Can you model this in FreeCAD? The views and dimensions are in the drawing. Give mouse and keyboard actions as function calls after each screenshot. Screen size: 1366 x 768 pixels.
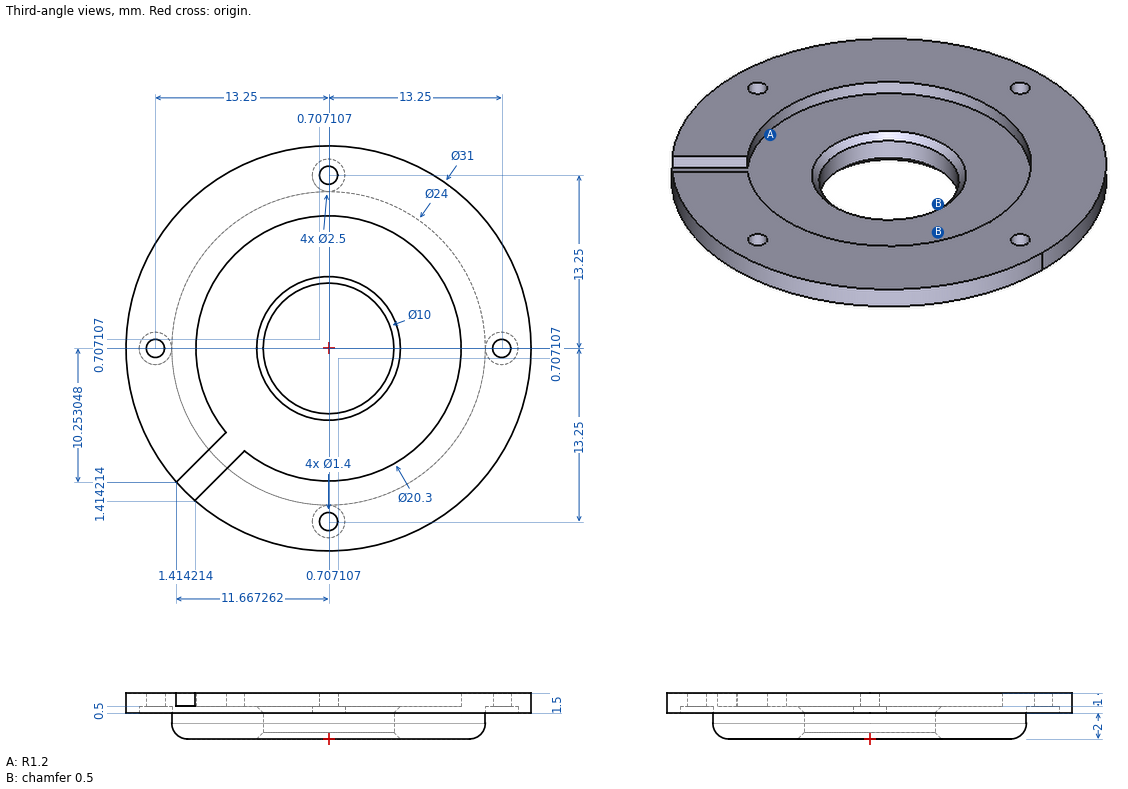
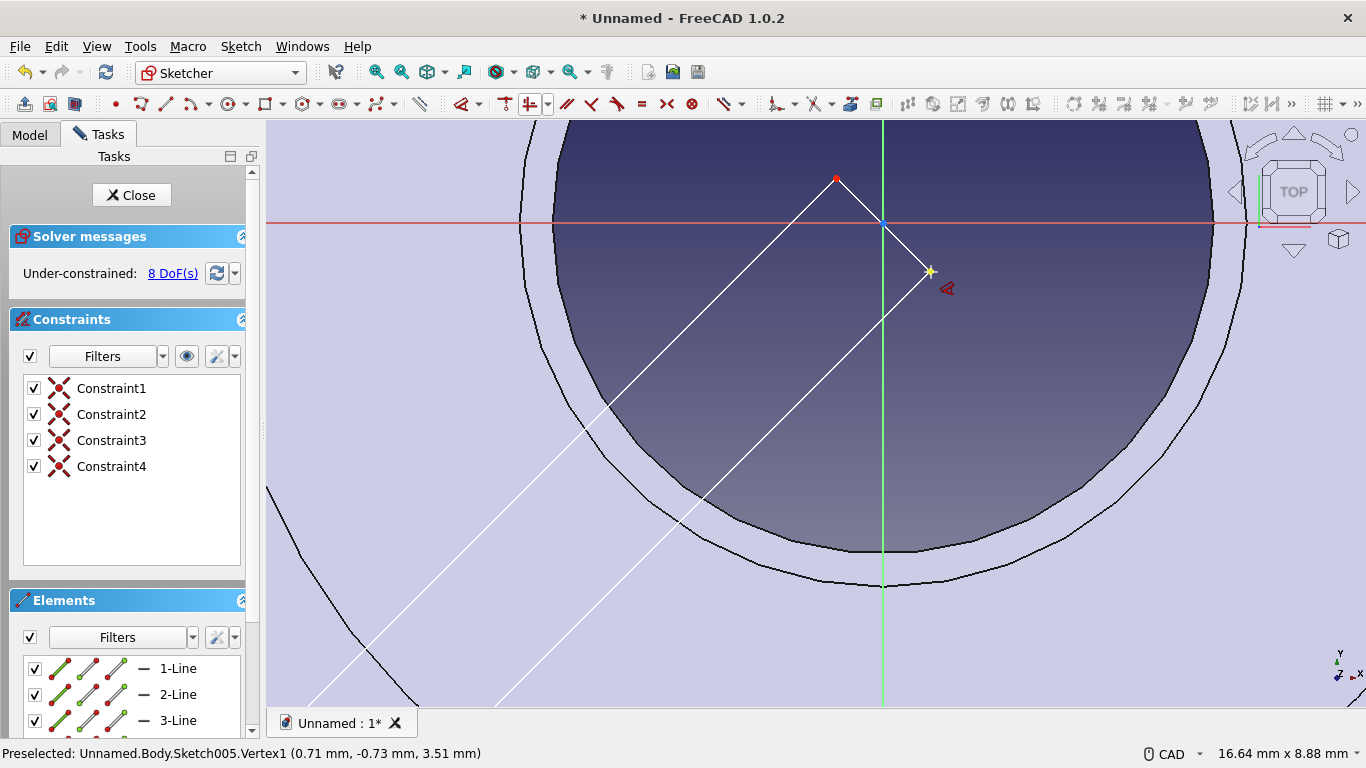
click(930, 272)
click(907, 189)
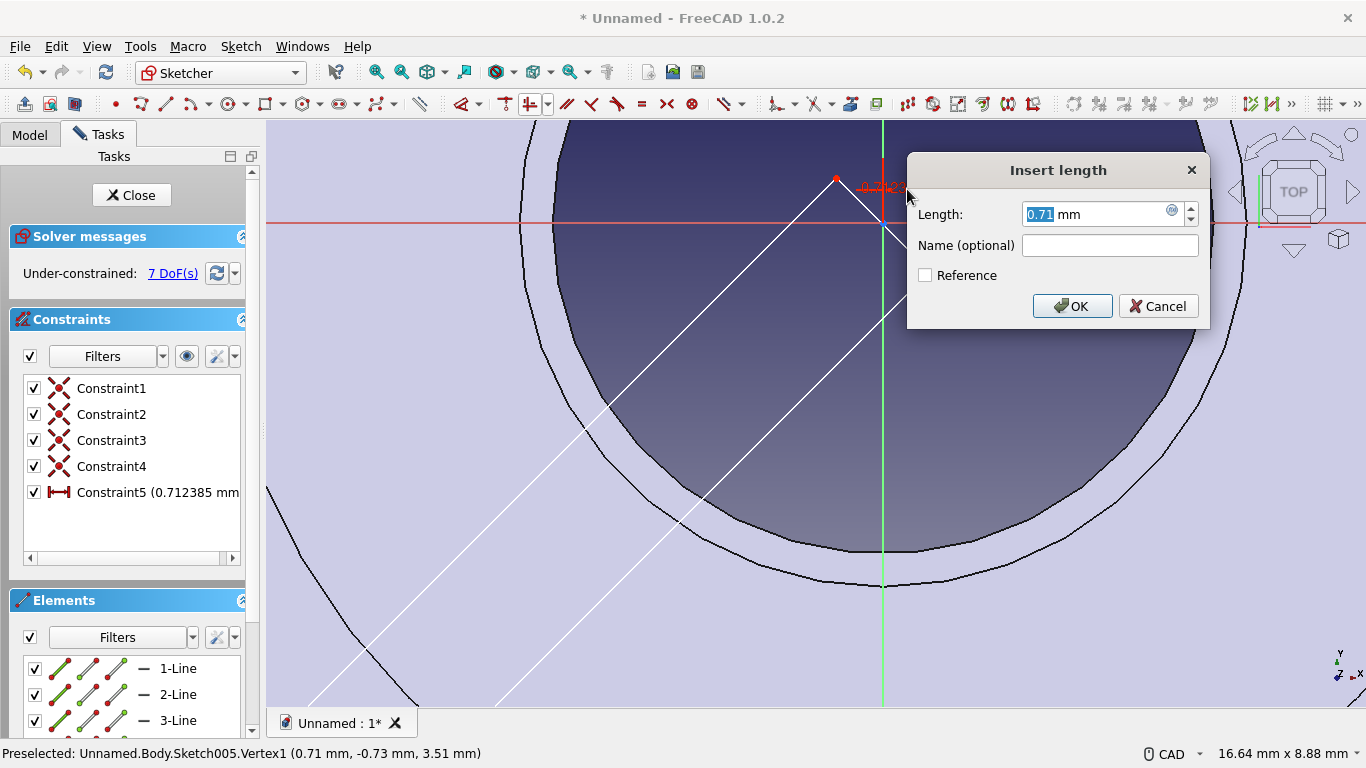
text(0.707107)
key(Return)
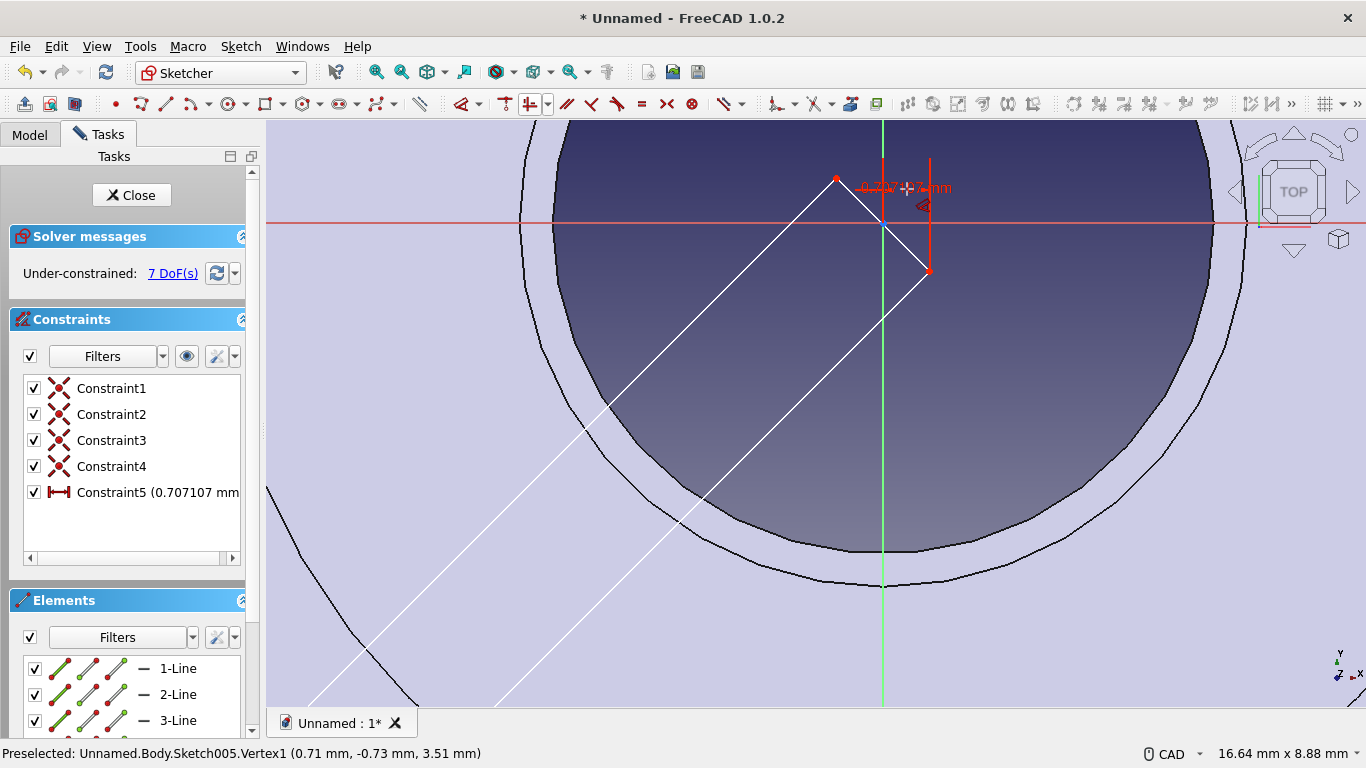
click(930, 272)
click(964, 247)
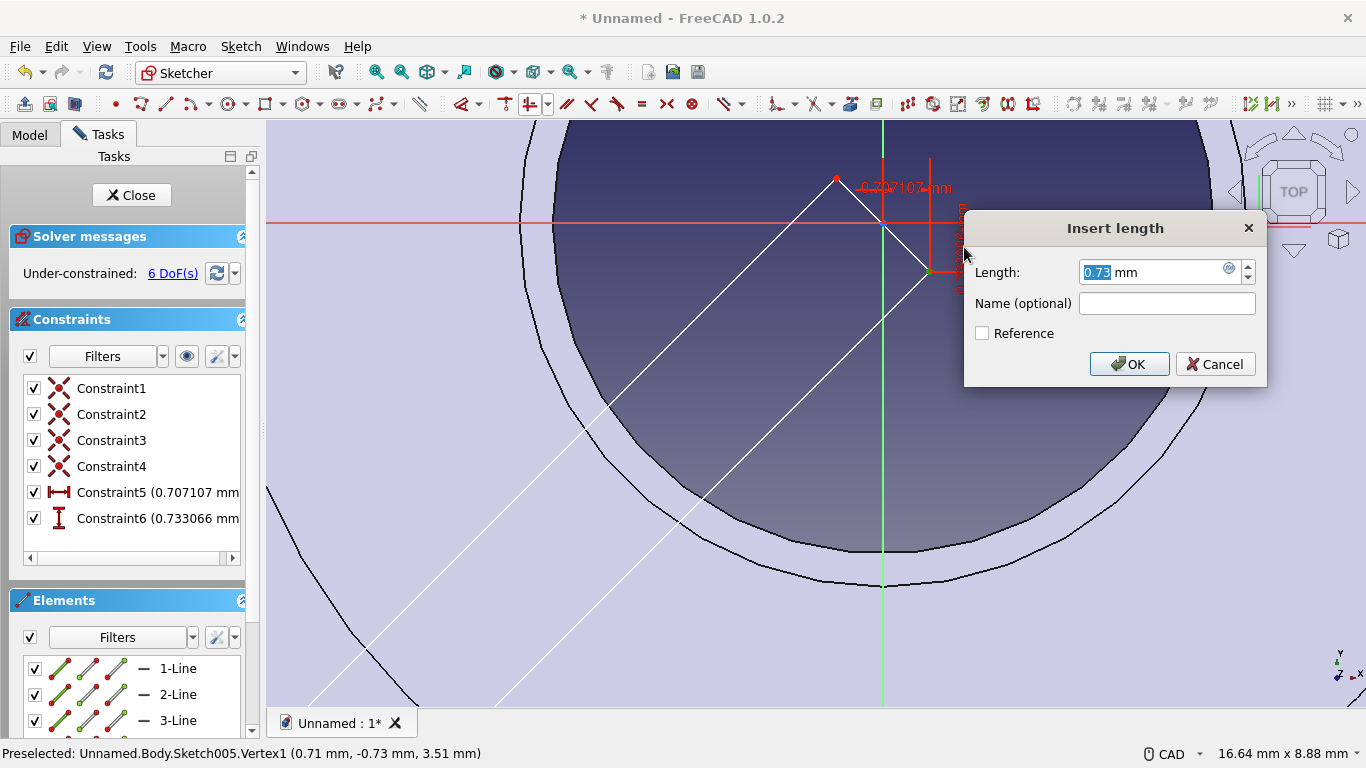
text(0.707107)
key(Return)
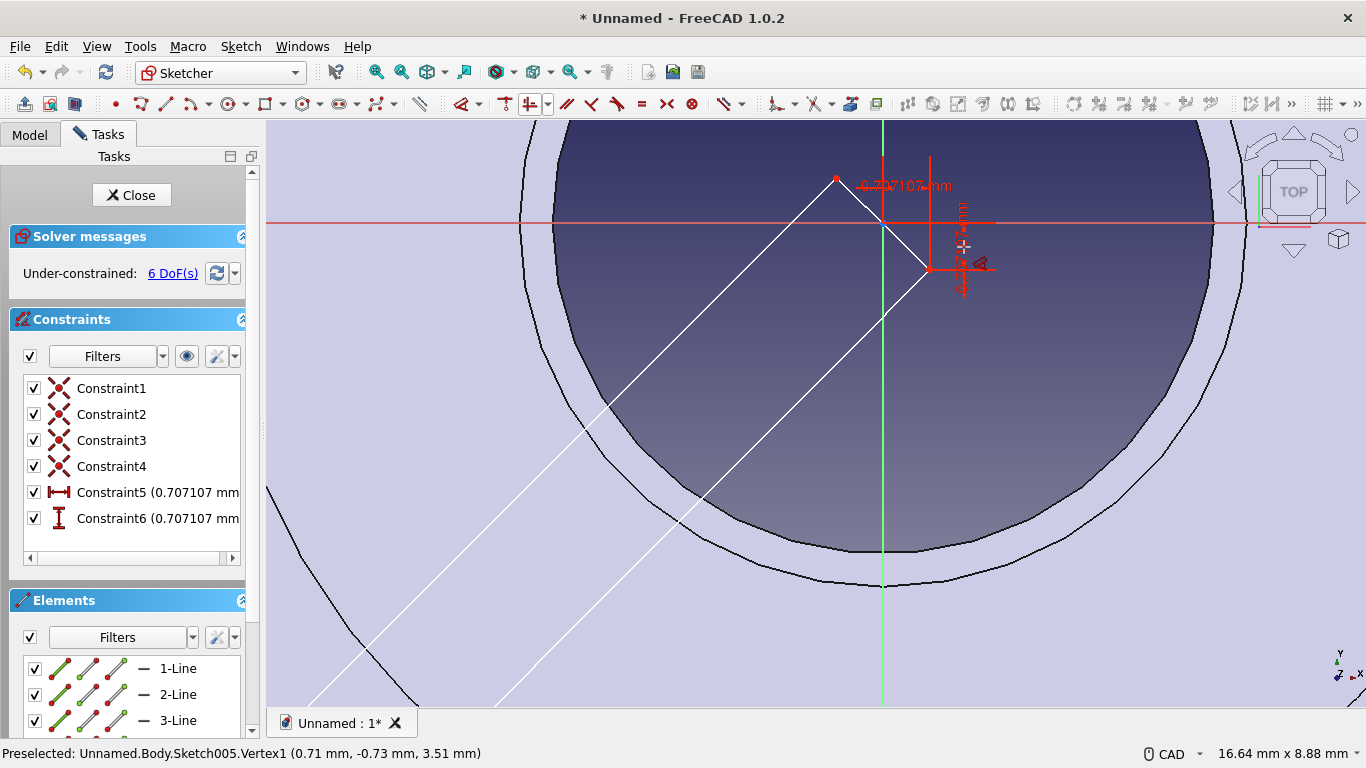
click(837, 178)
click(860, 257)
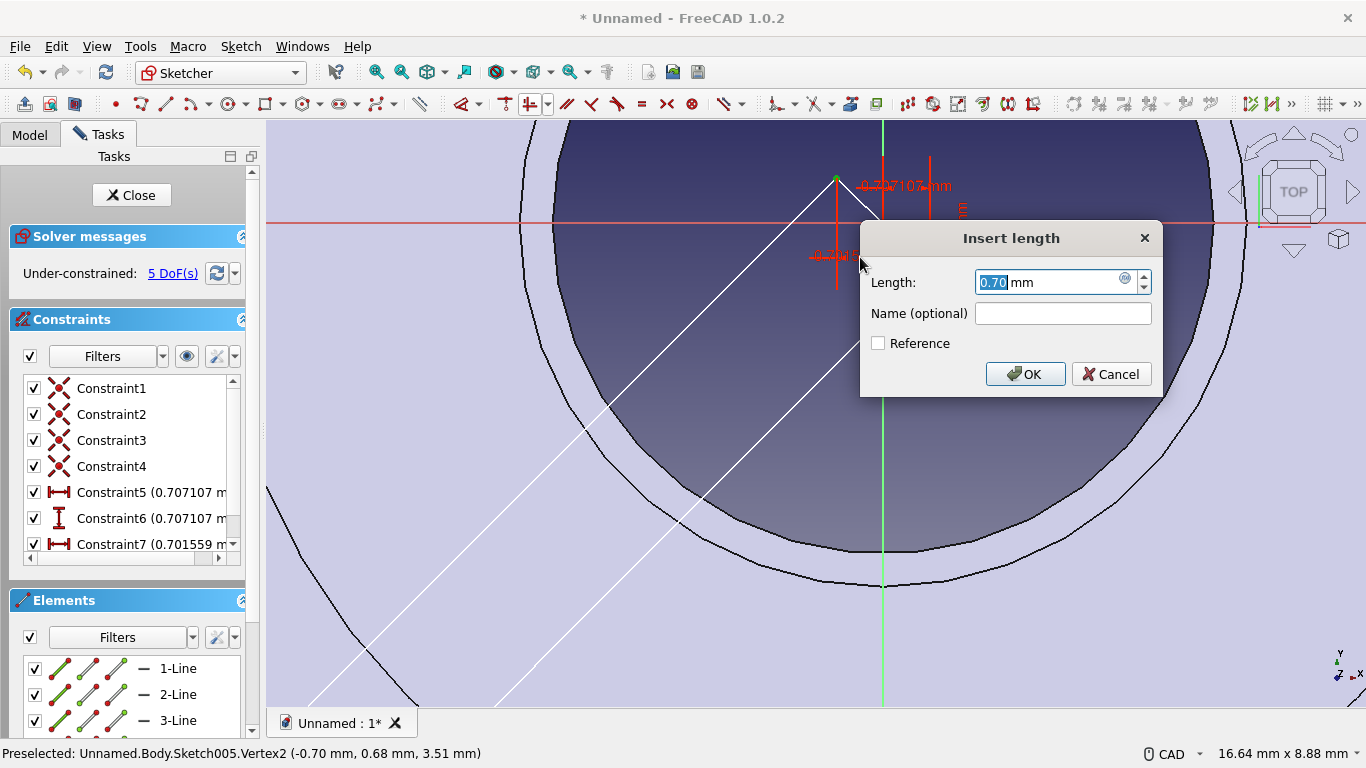
text(0.707107)
key(Return)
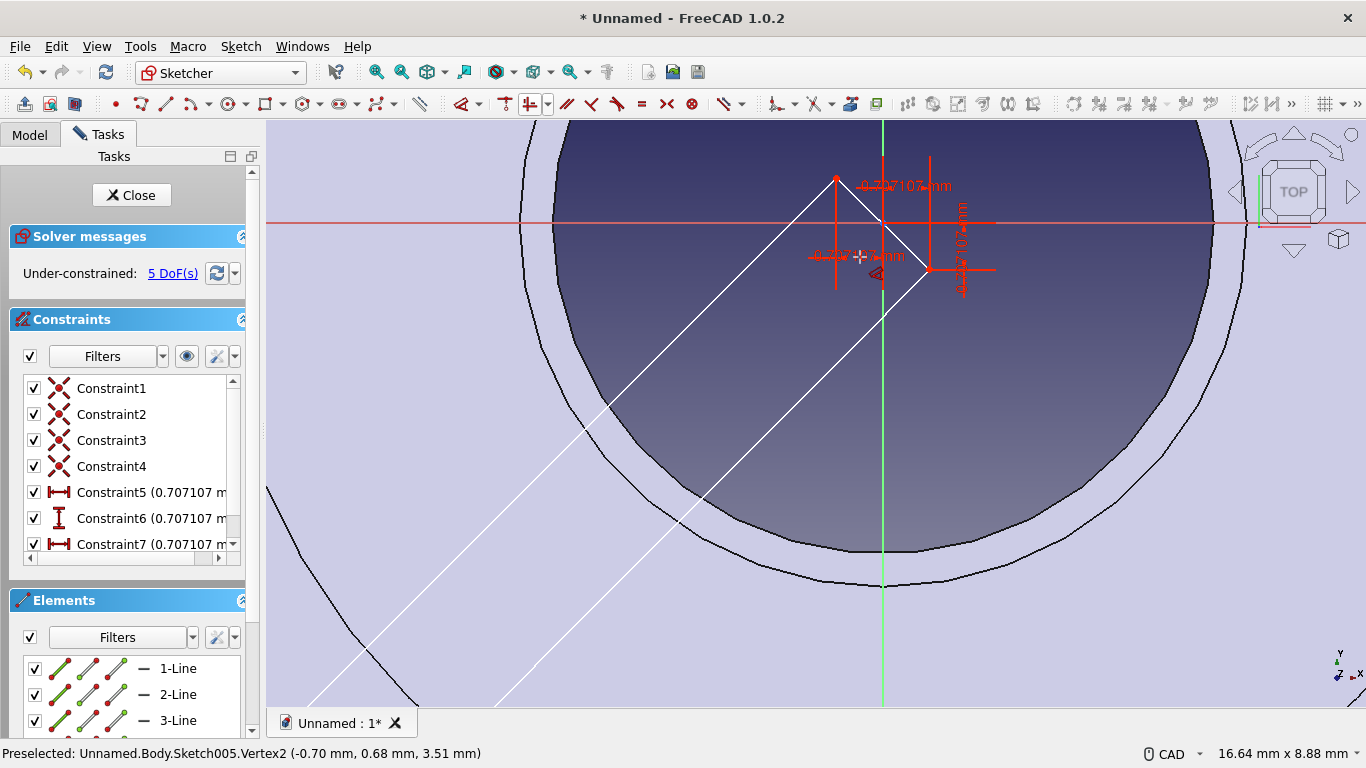
click(836, 178)
click(802, 190)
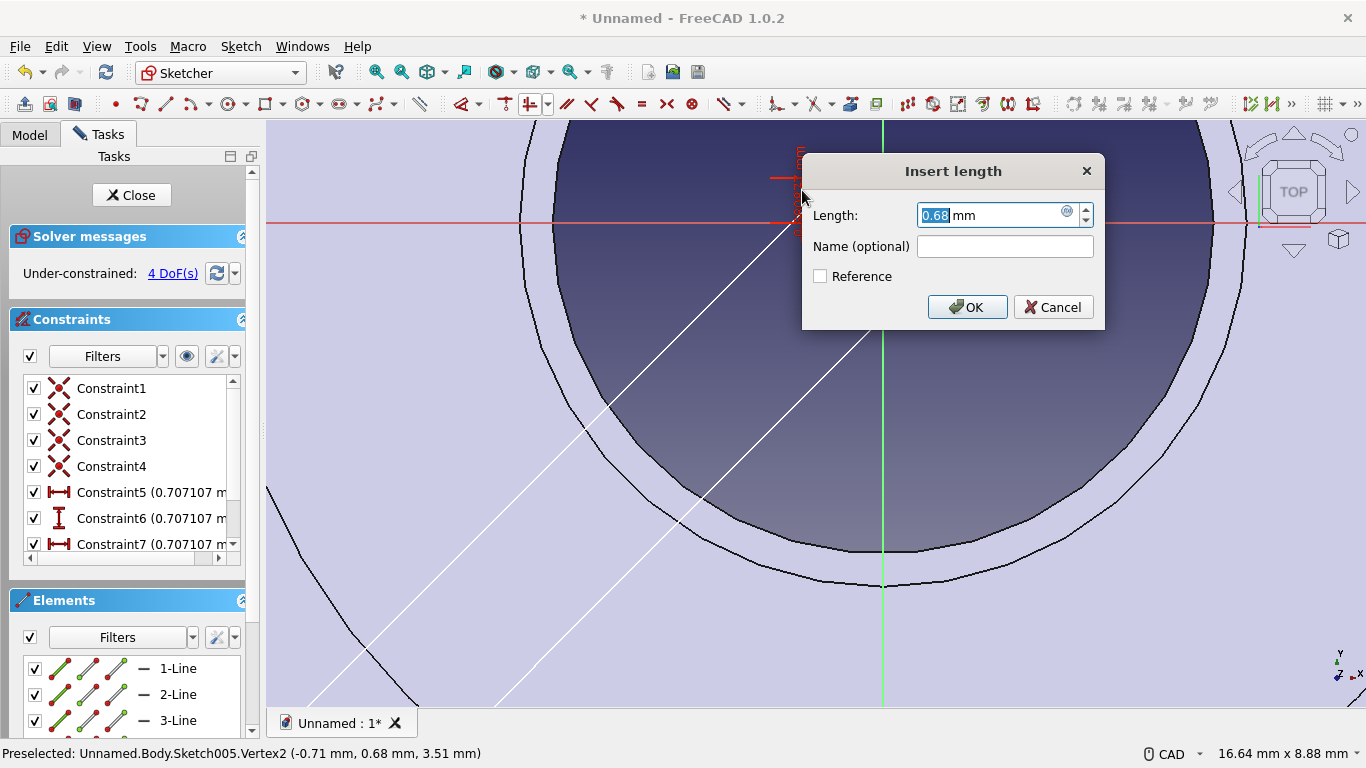
text(0.707107)
key(Return)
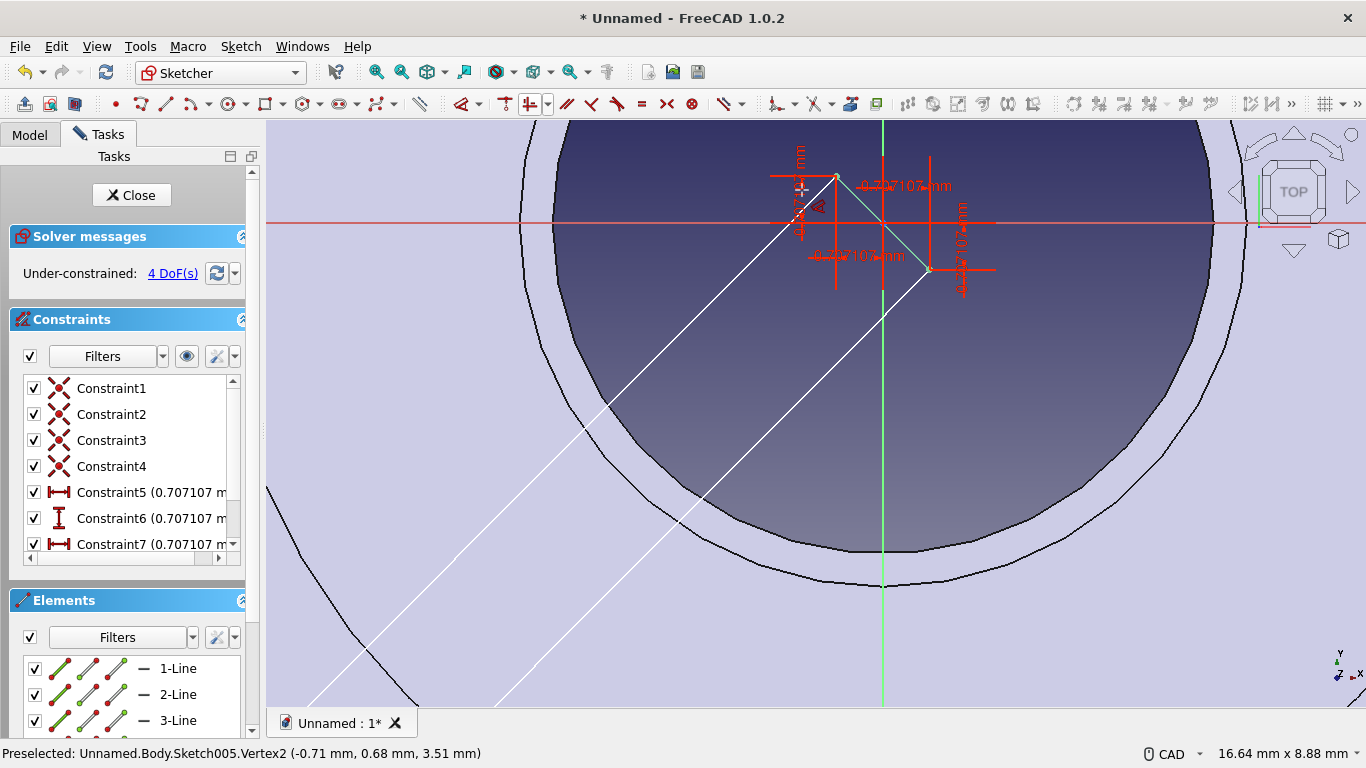
scroll(932, 273, down, 4)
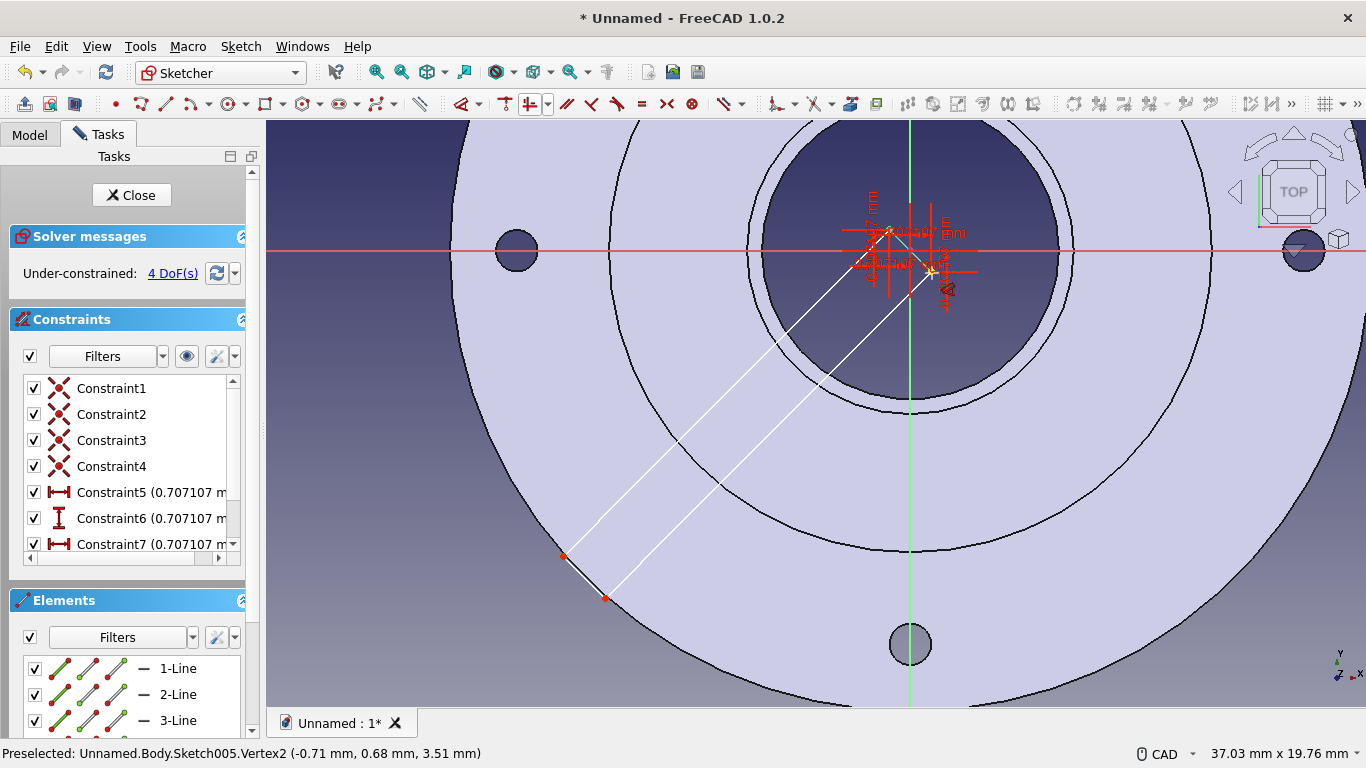
click(576, 569)
click(585, 633)